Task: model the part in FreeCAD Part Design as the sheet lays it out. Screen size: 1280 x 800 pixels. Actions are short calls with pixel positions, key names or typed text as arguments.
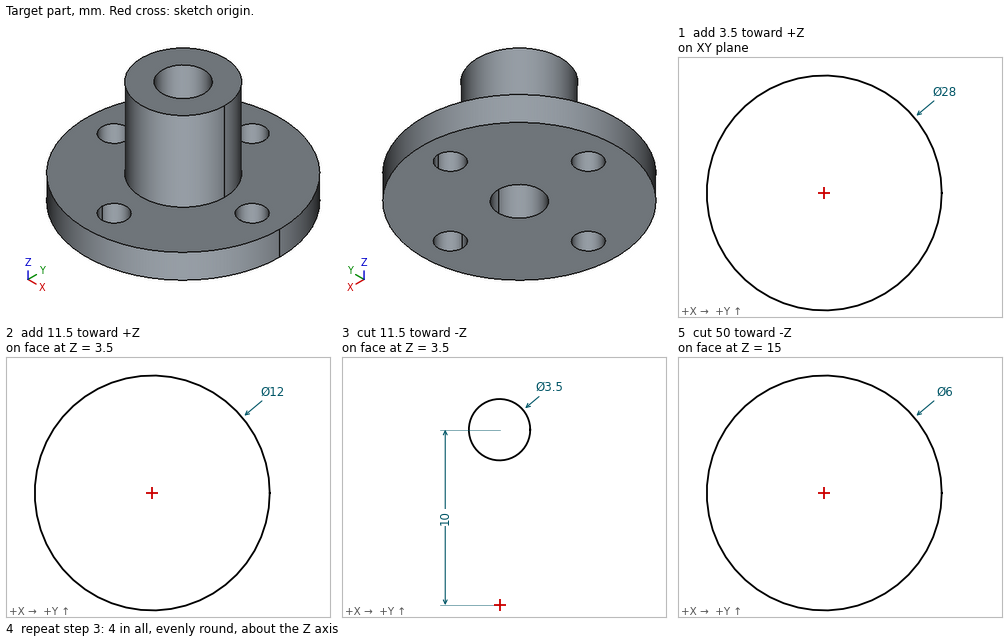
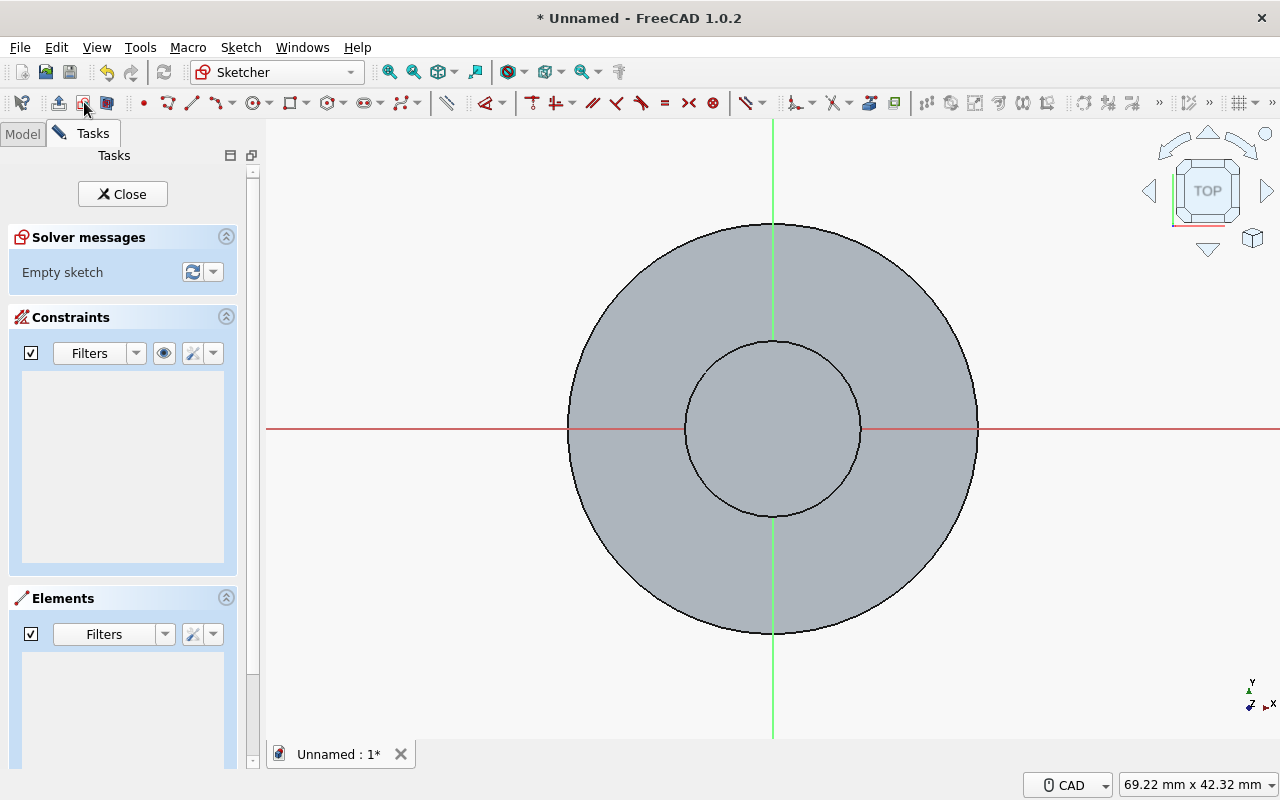
key(q)
key(s)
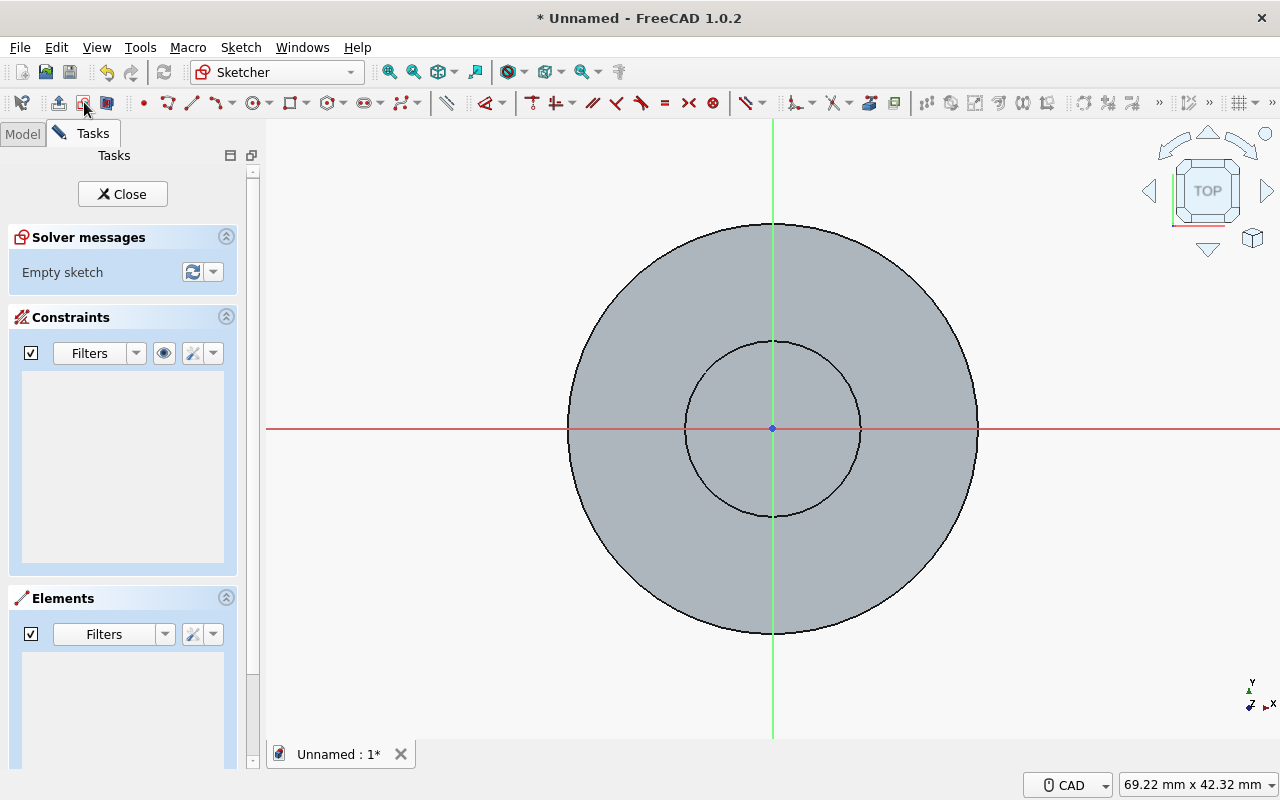
scroll(784, 260, up, 10)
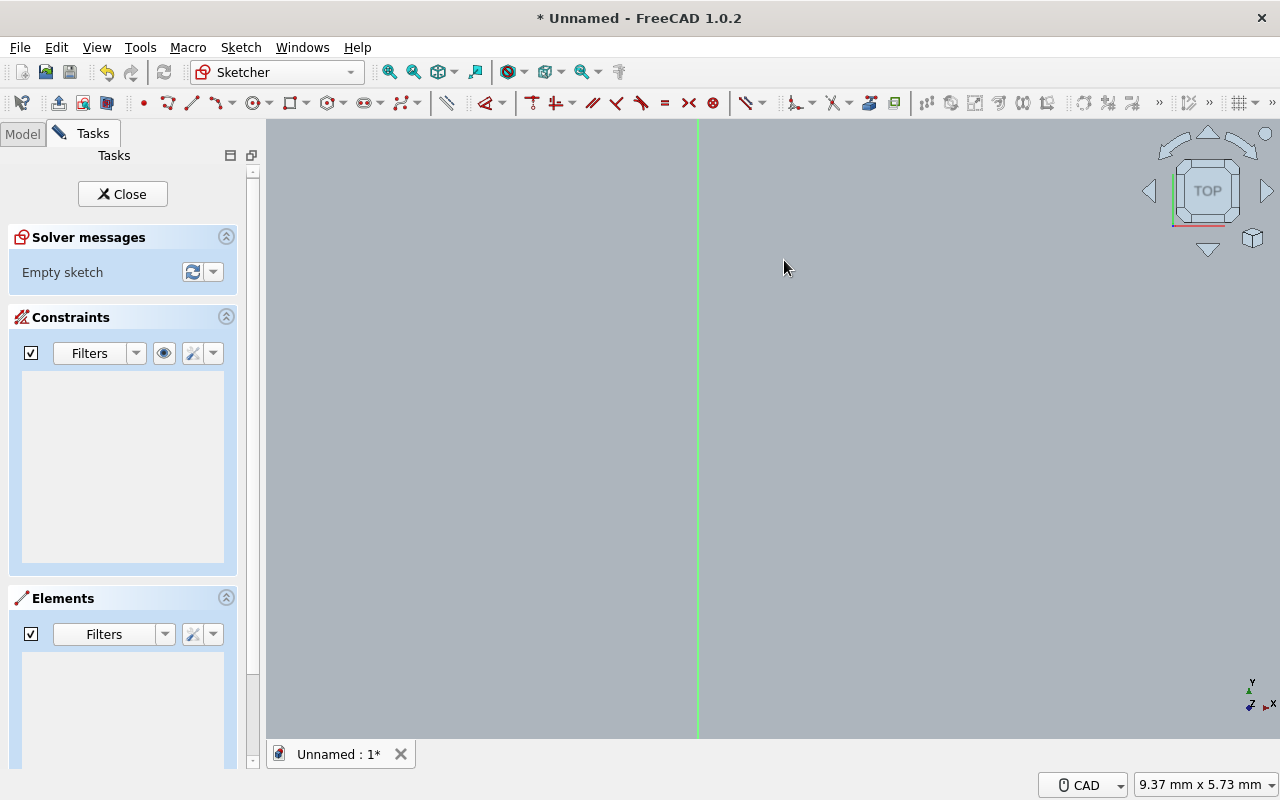
key(g)
key(c)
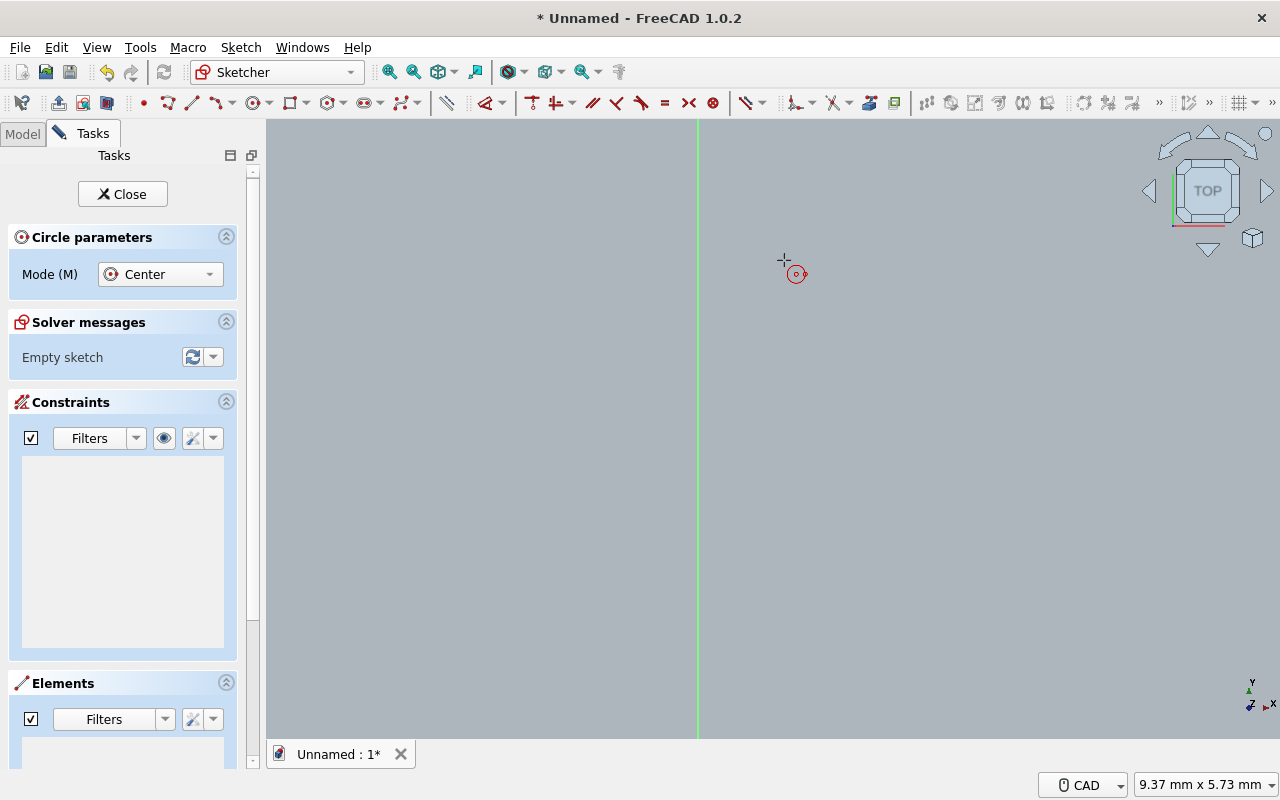
click(698, 425)
click(832, 291)
key(Escape)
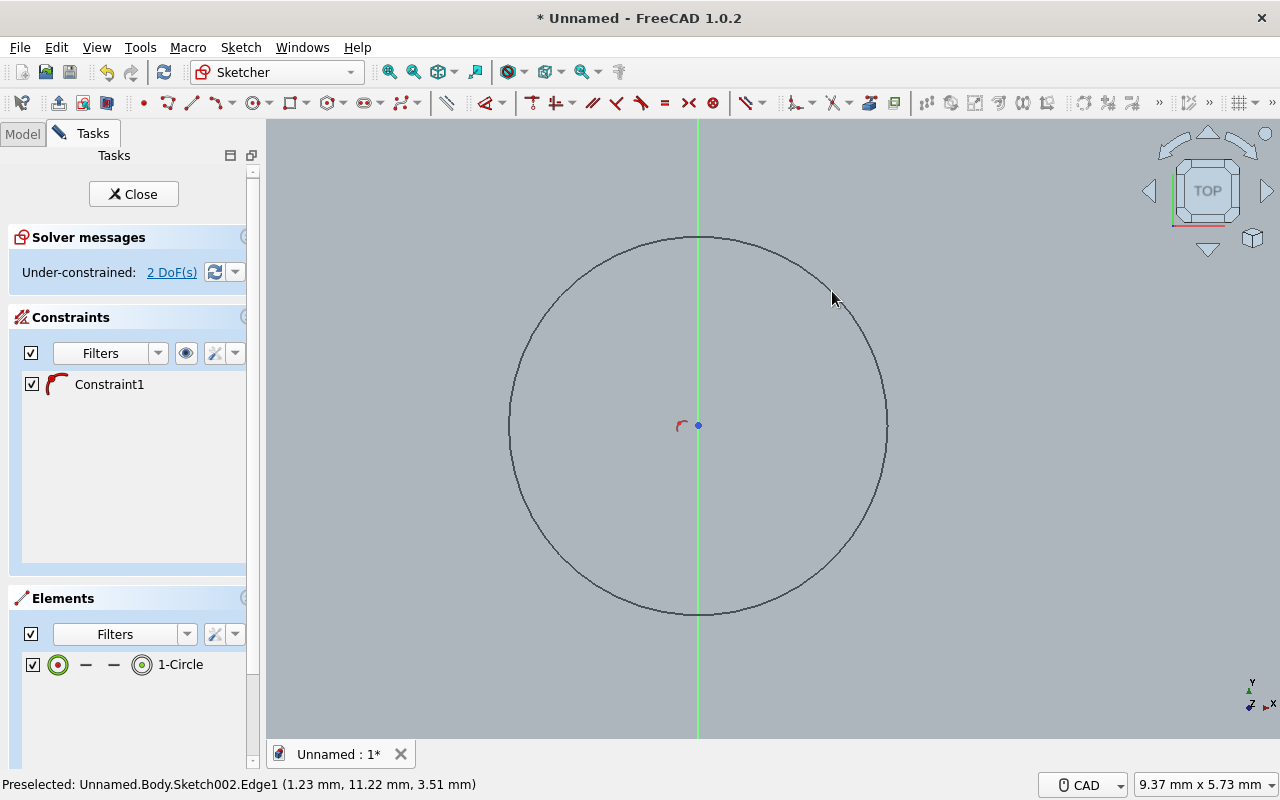
key(d)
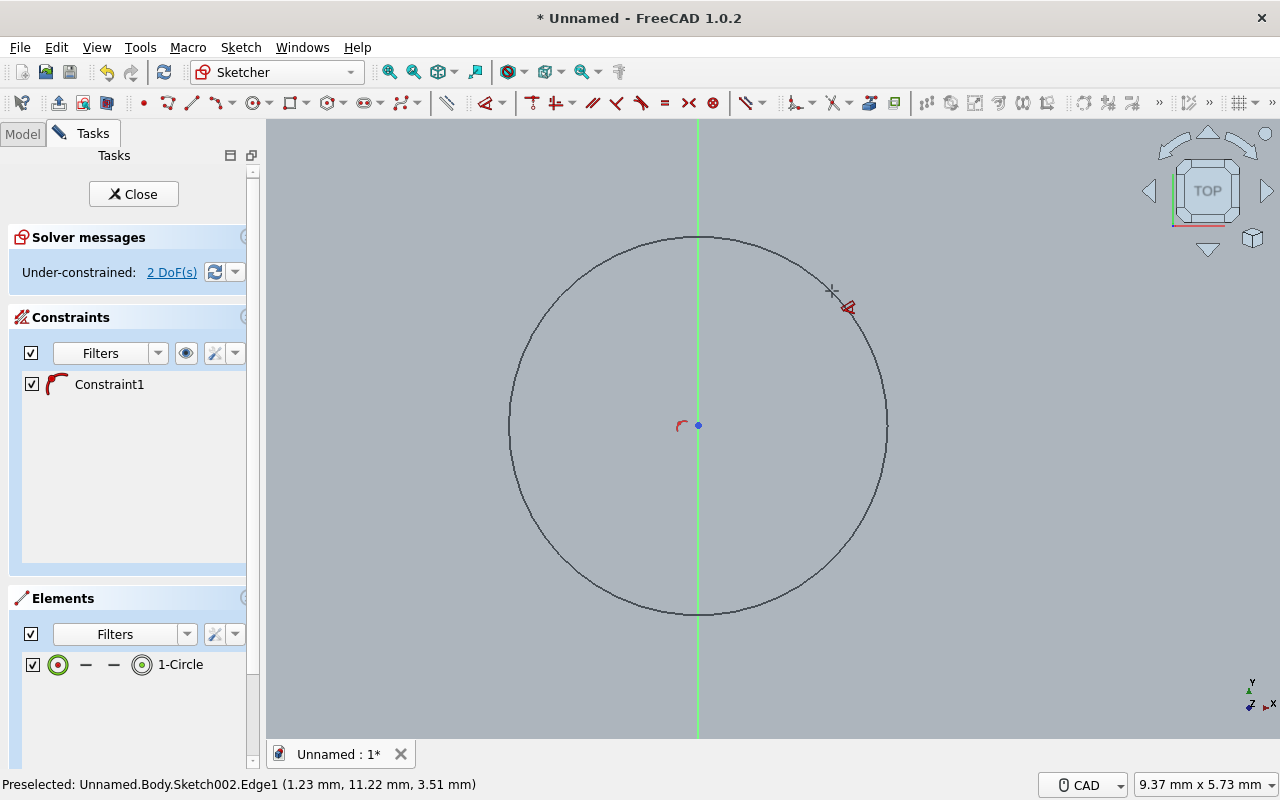
click(832, 292)
click(855, 269)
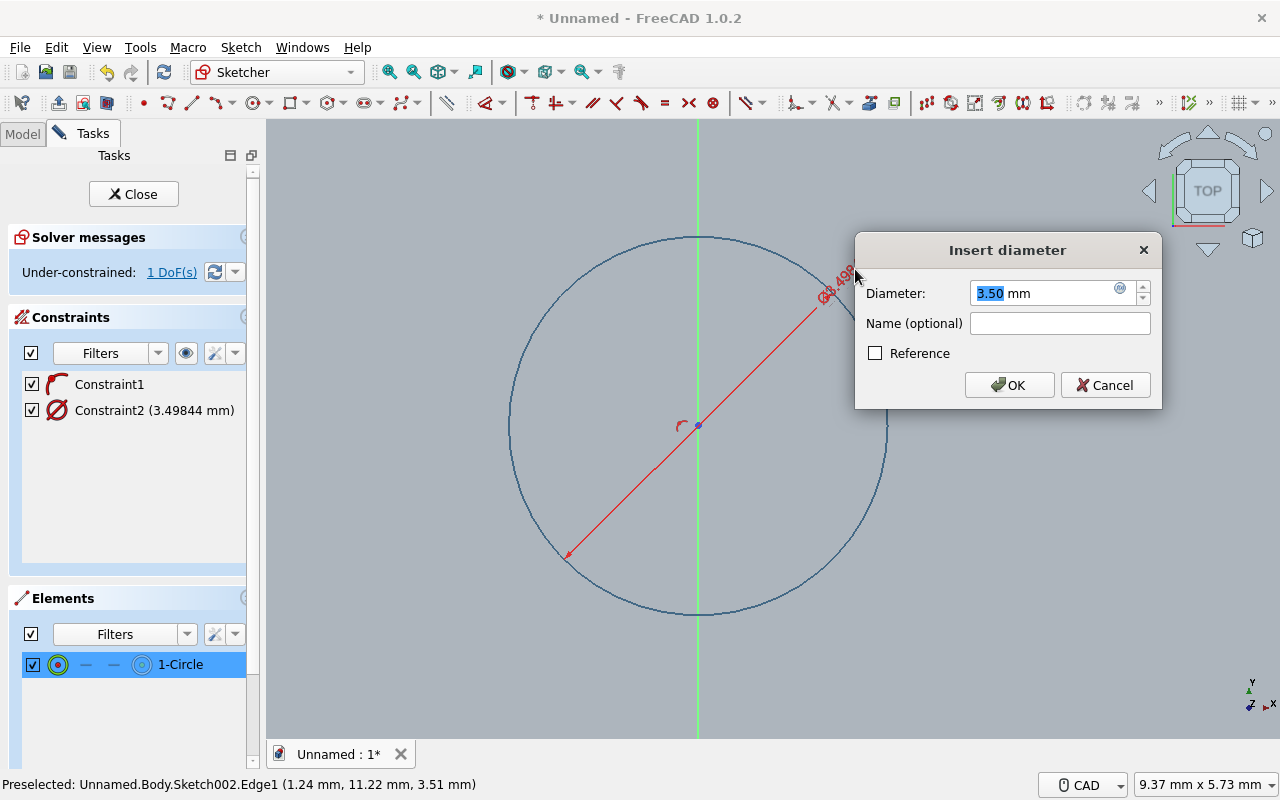
text(3.5)
key(Return)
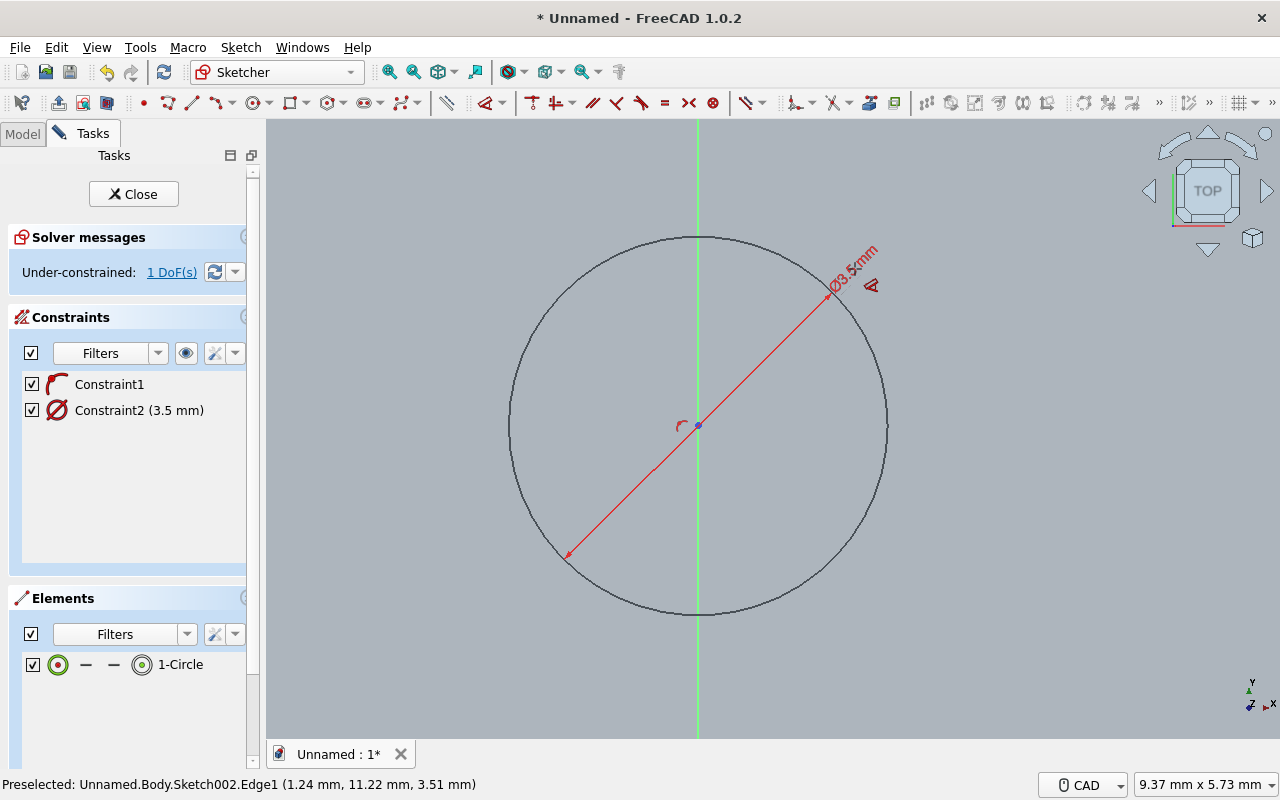
click(698, 426)
click(732, 569)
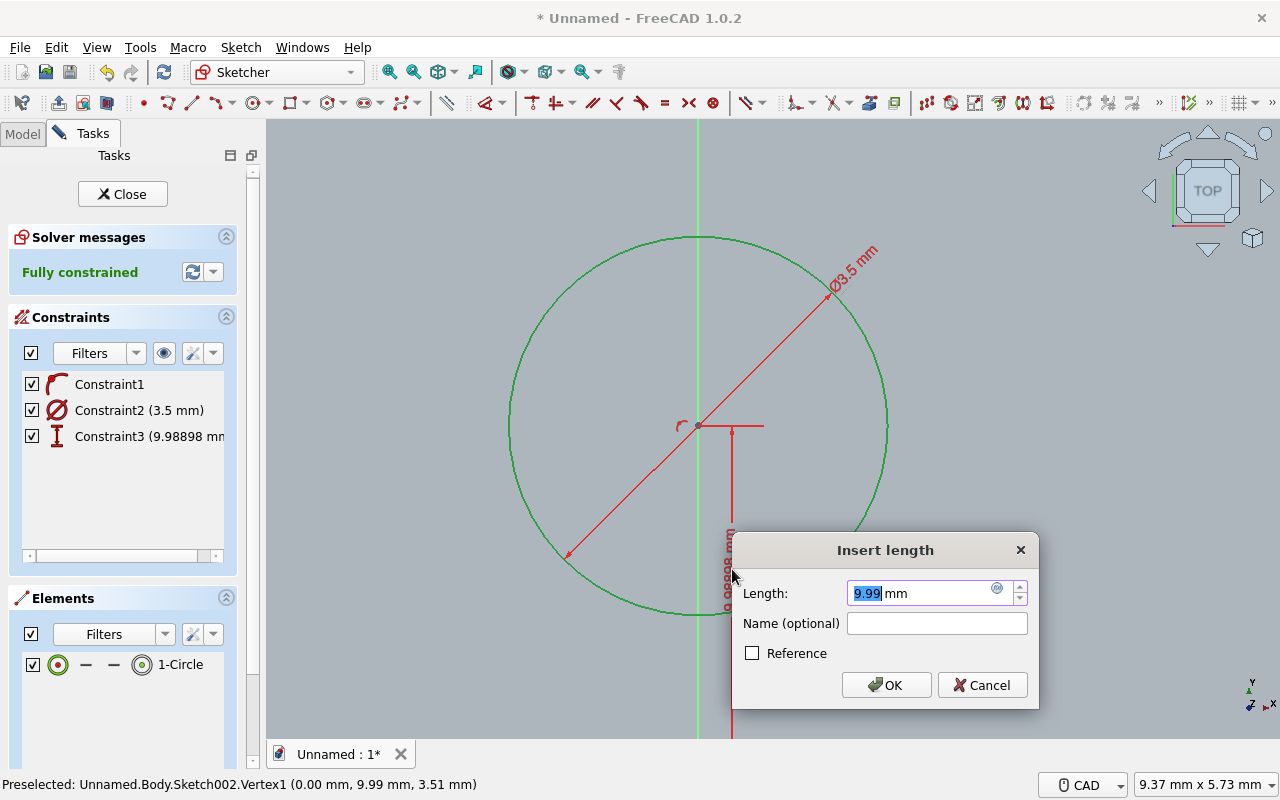
text(10)
key(Return)
key(Escape)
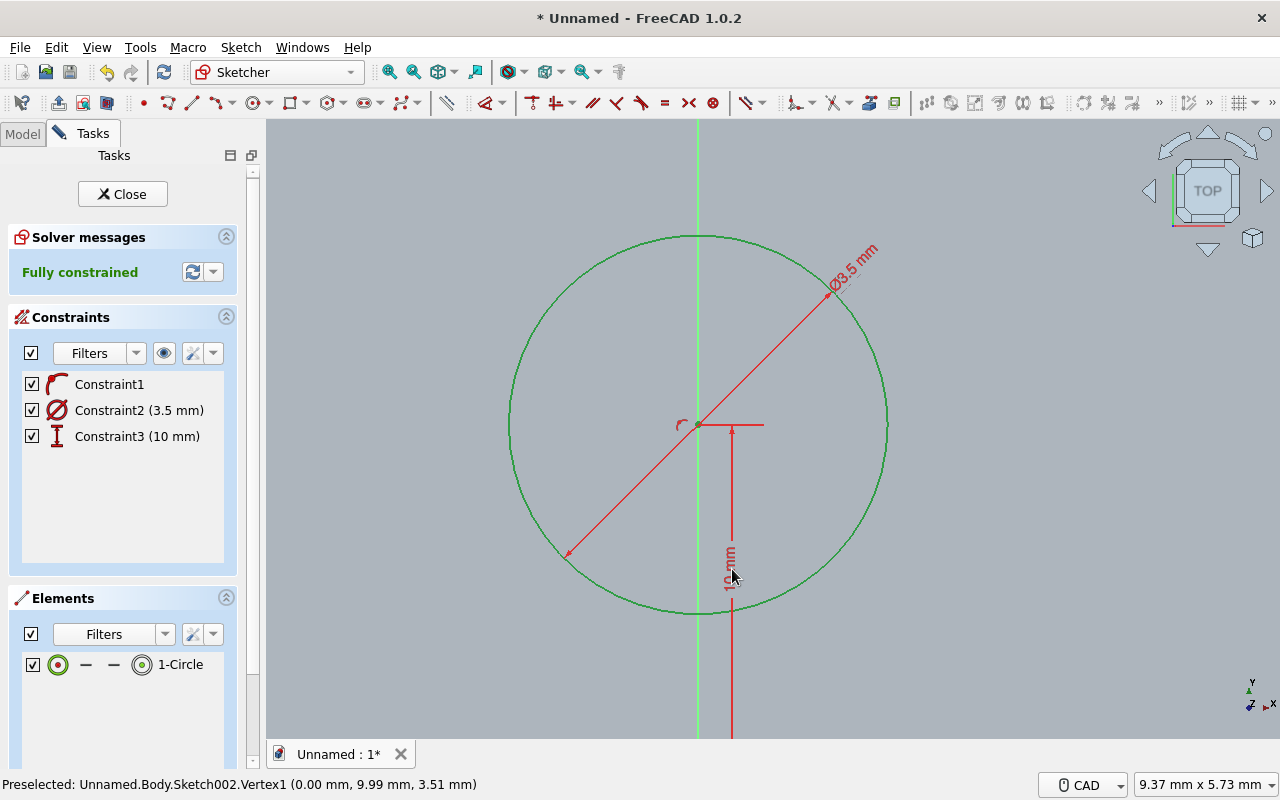
click(123, 194)